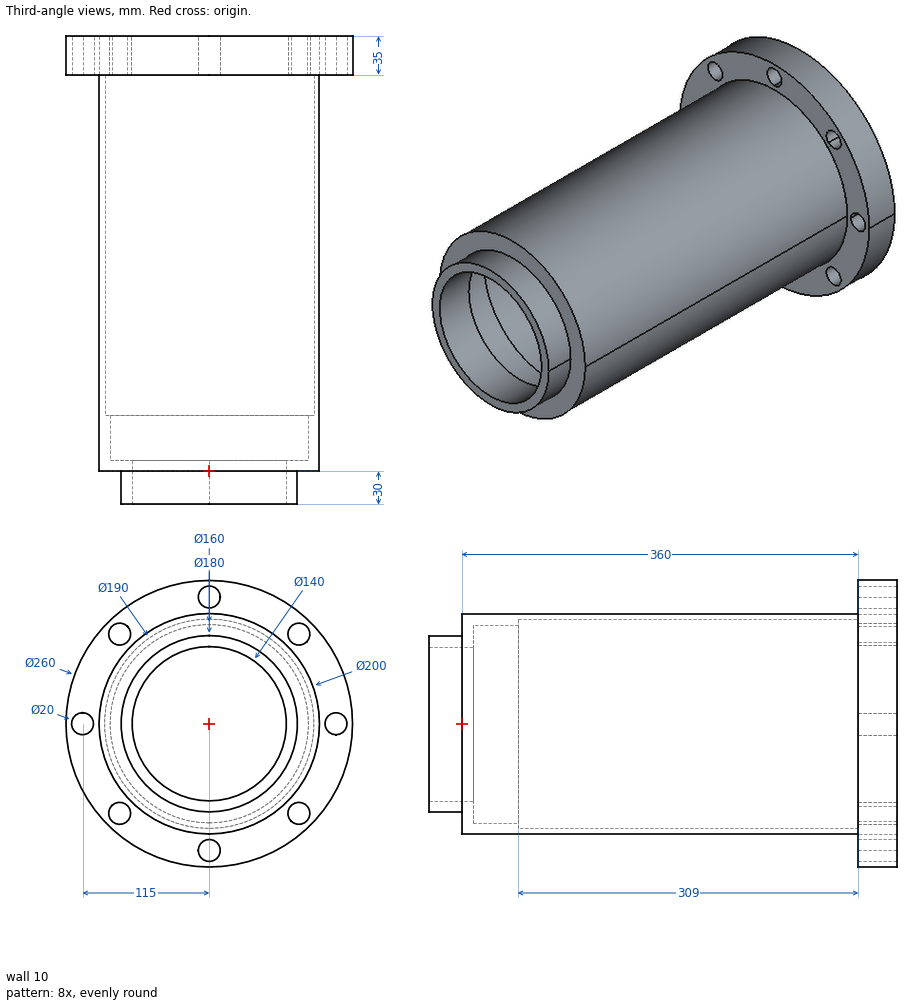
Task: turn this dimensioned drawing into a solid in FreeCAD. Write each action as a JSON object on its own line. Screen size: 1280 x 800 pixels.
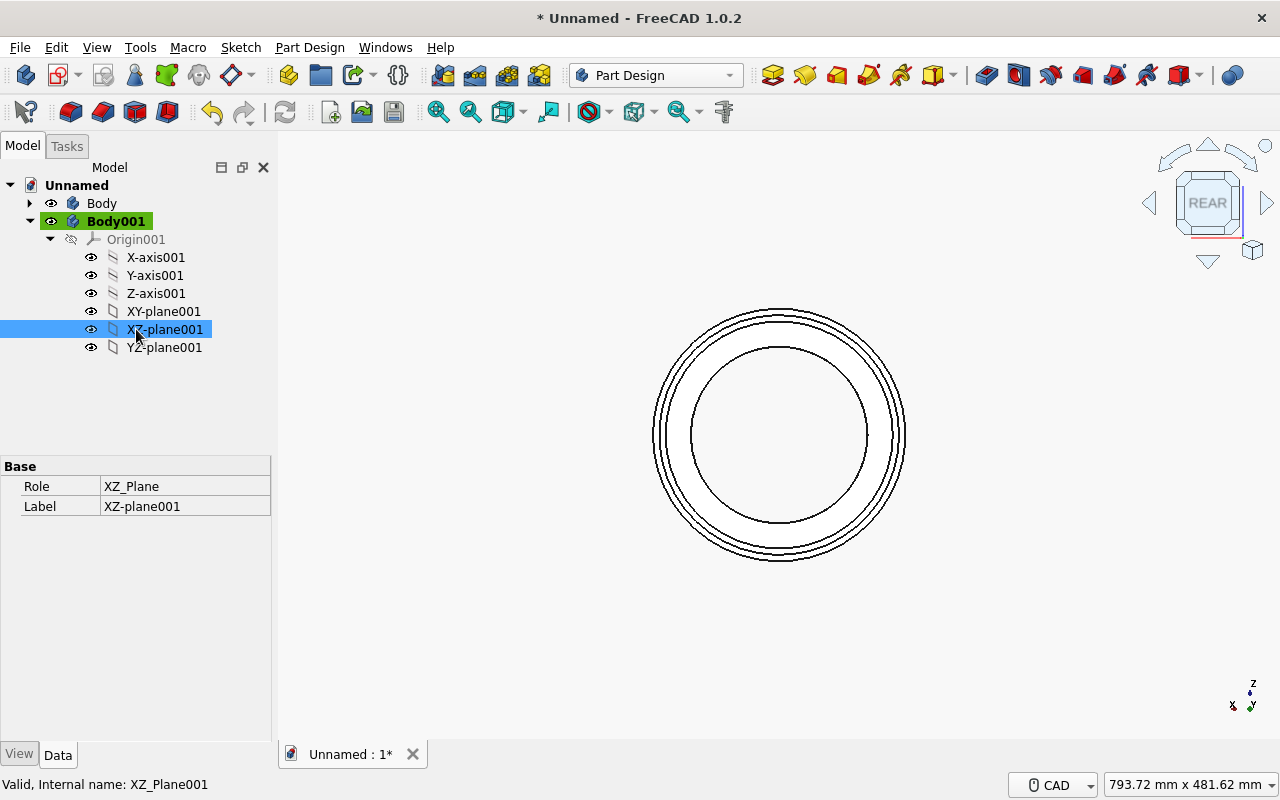
{"action": "left_click", "coordinate": [232, 76]}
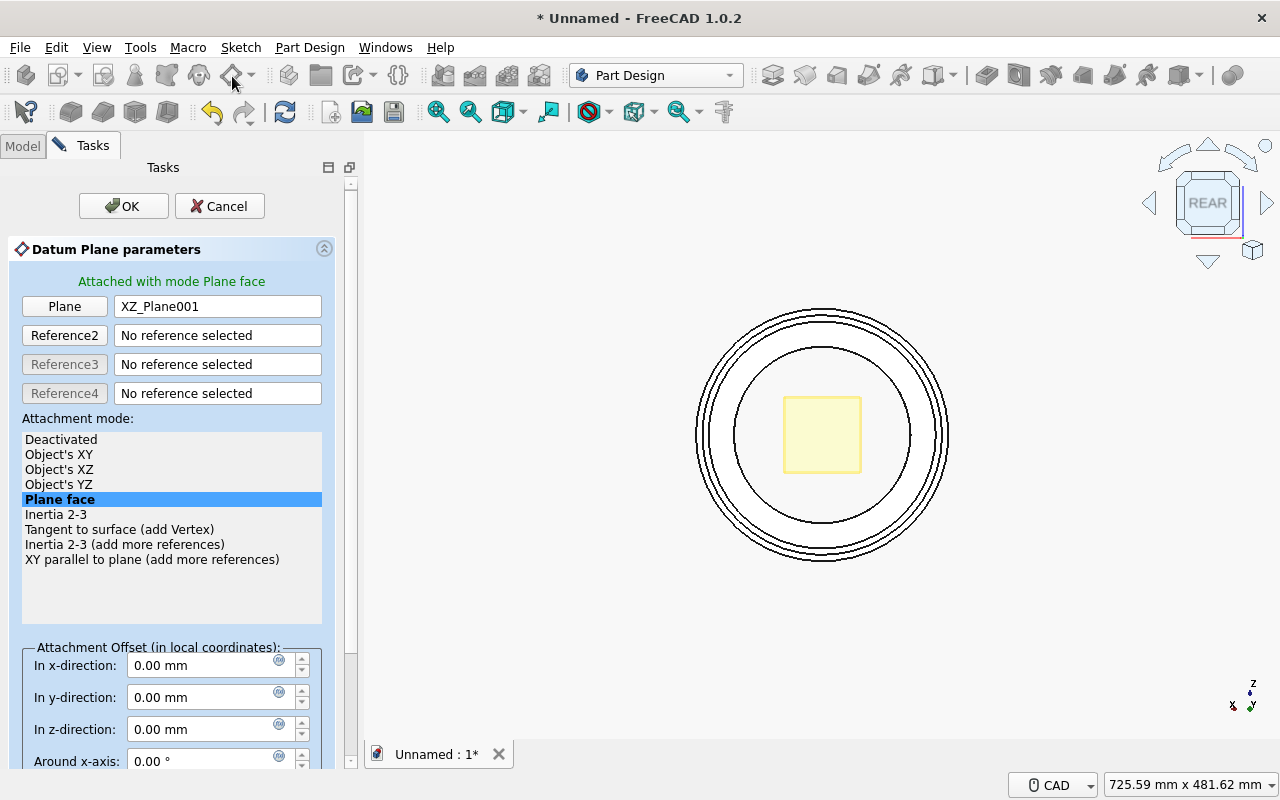
{"action": "triple_click", "coordinate": [210, 729]}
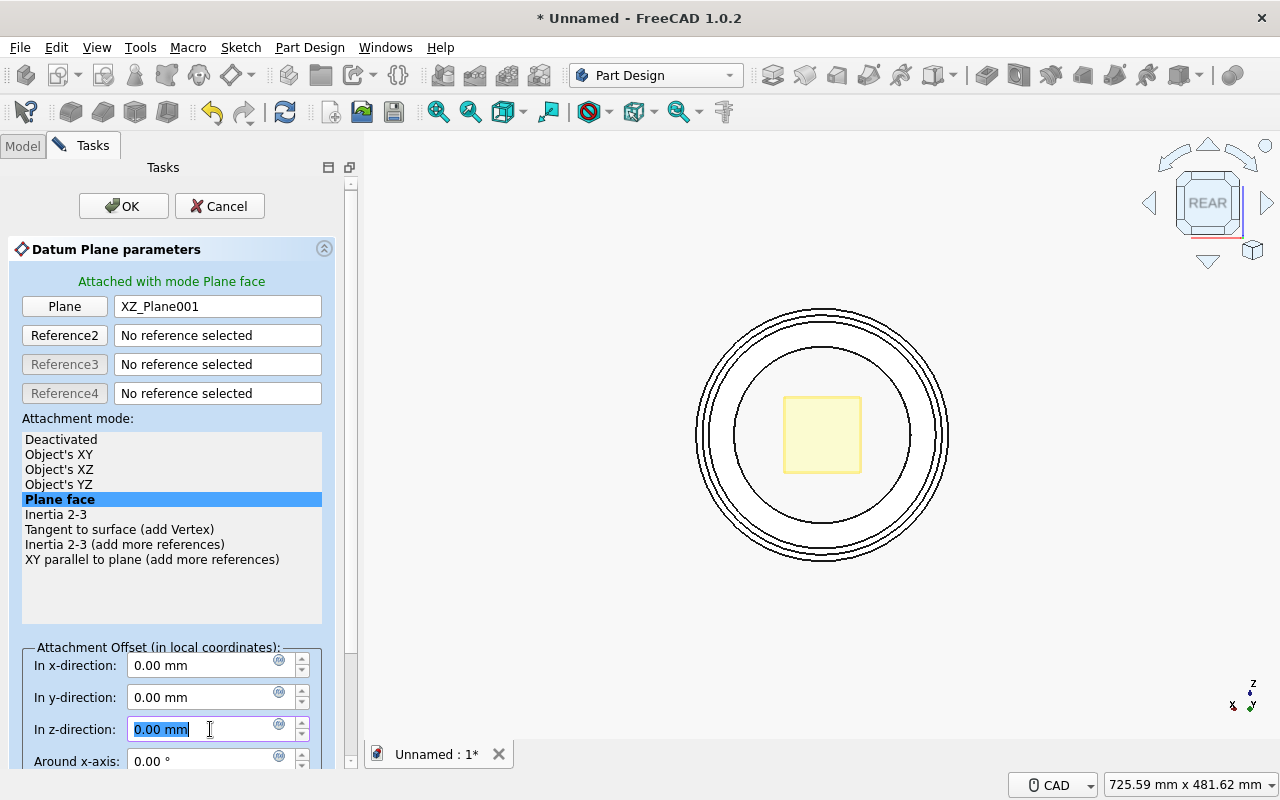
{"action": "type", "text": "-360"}
{"action": "key", "text": "Tab"}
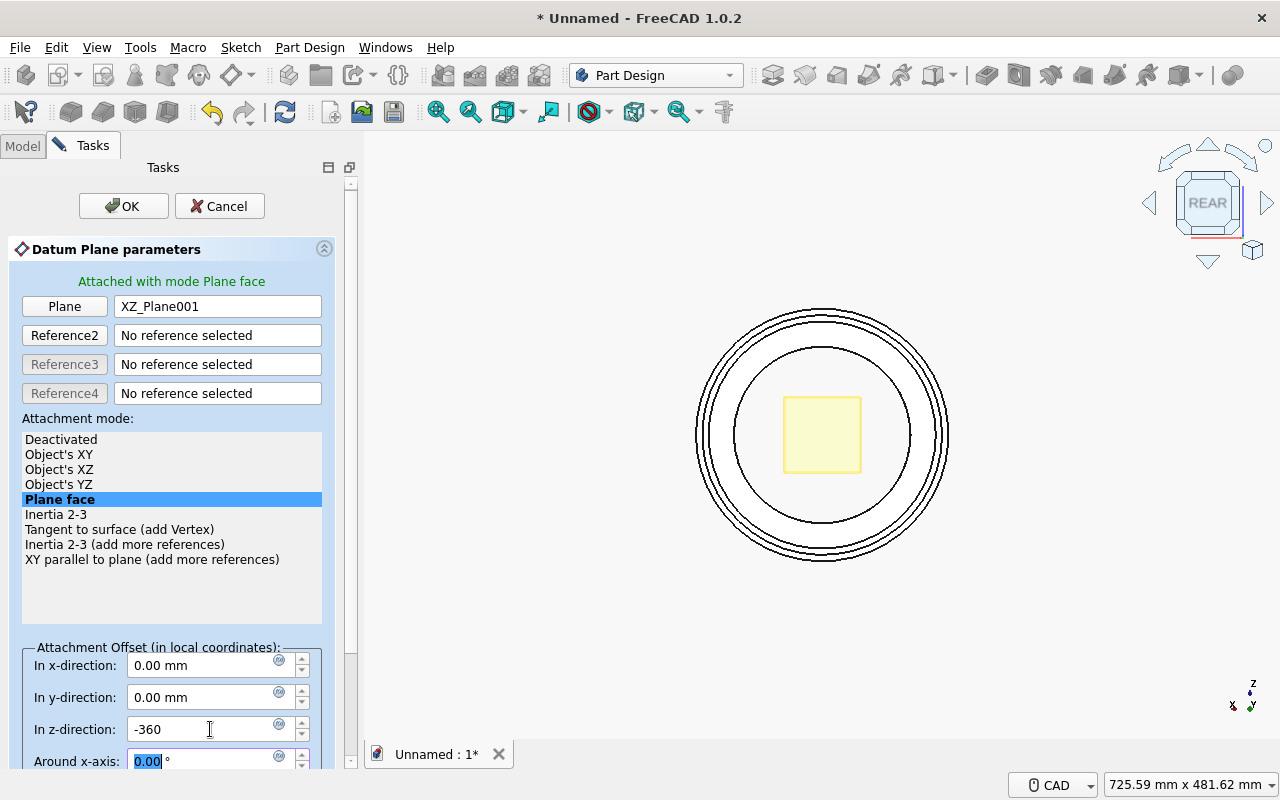
{"action": "left_click", "coordinate": [124, 206]}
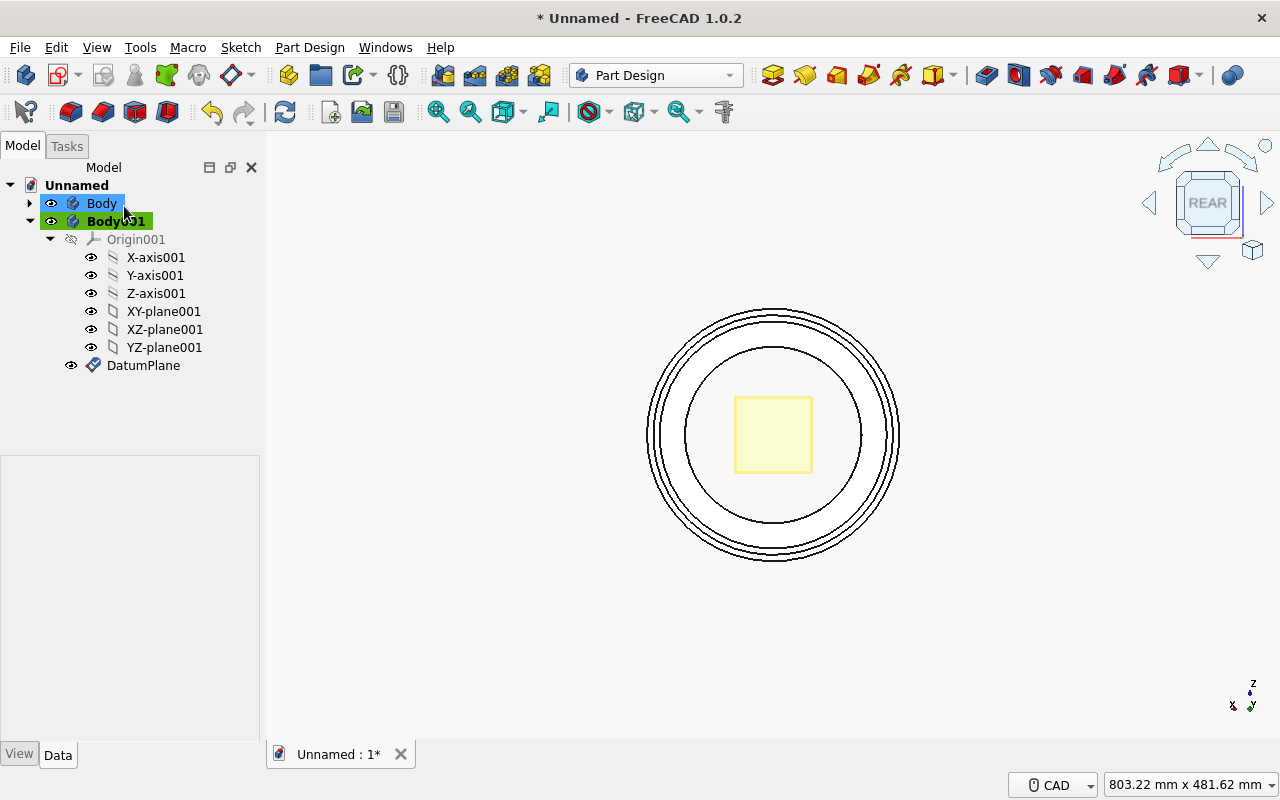
{"action": "left_click", "coordinate": [116, 365]}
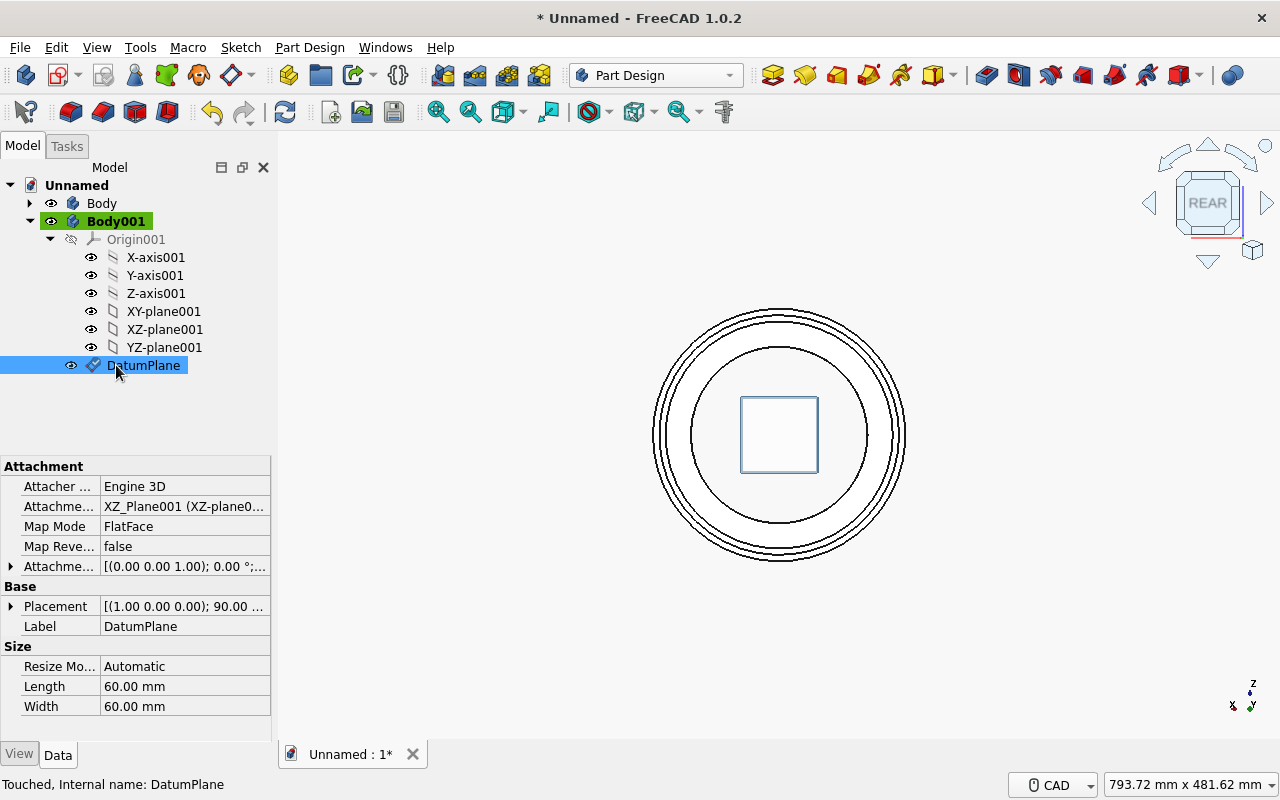
{"action": "left_click", "coordinate": [58, 76]}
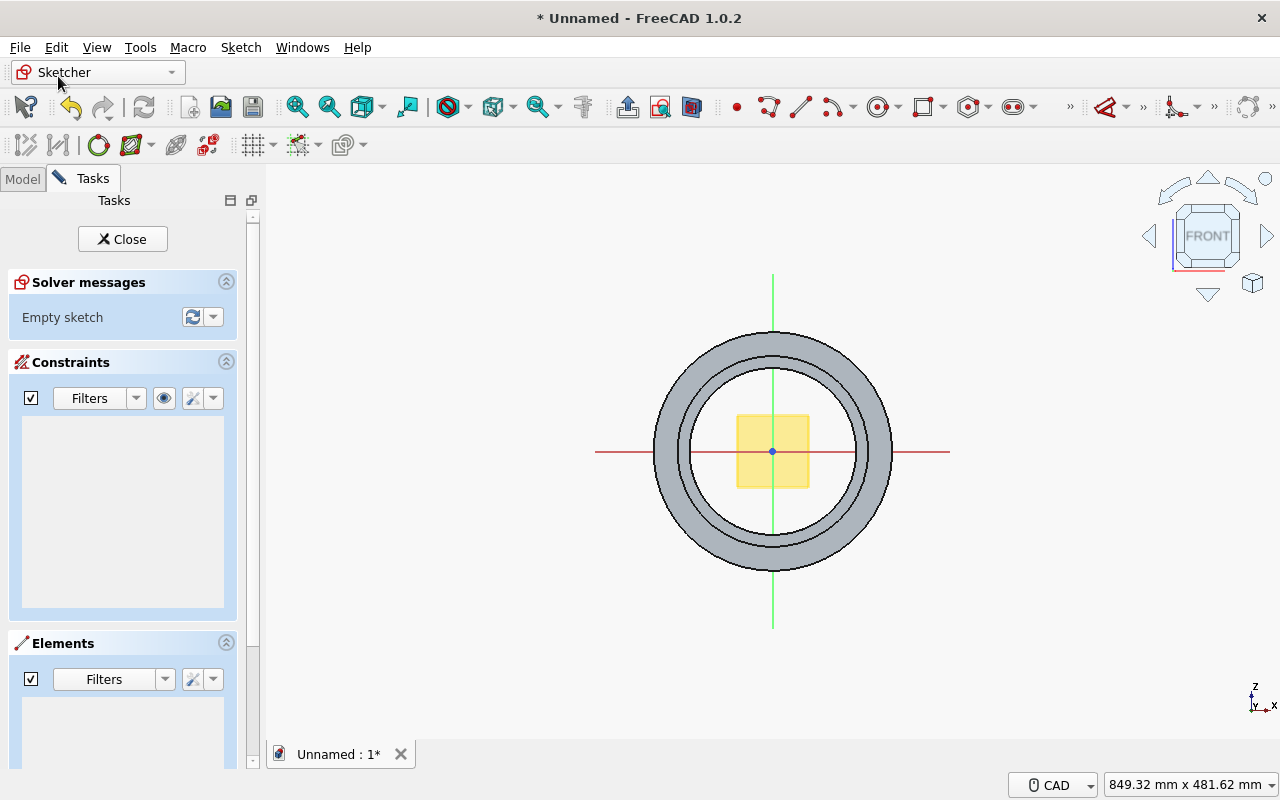
{"action": "left_click", "coordinate": [878, 108]}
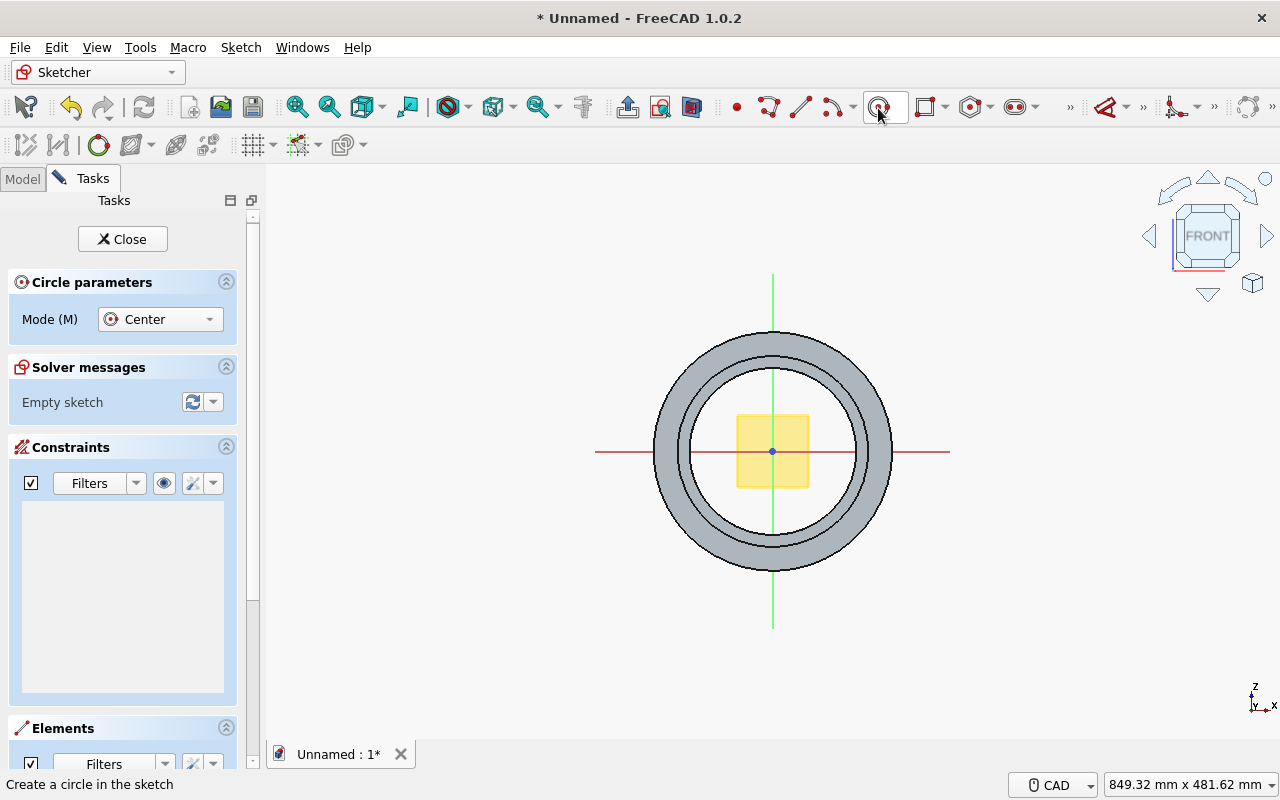
{"action": "left_click", "coordinate": [773, 452]}
{"action": "left_click", "coordinate": [883, 342]}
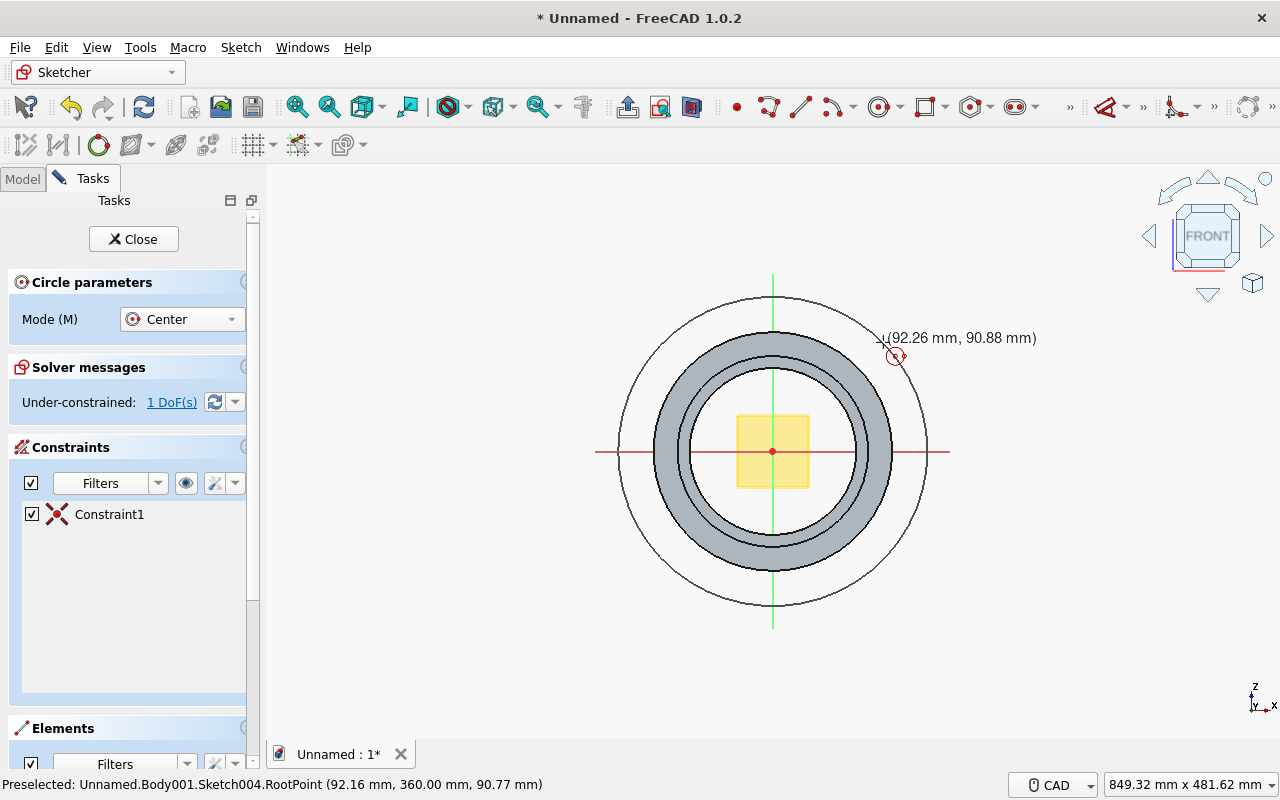
{"action": "left_click", "coordinate": [773, 452]}
{"action": "left_click", "coordinate": [857, 367]}
{"action": "key", "text": "Escape"}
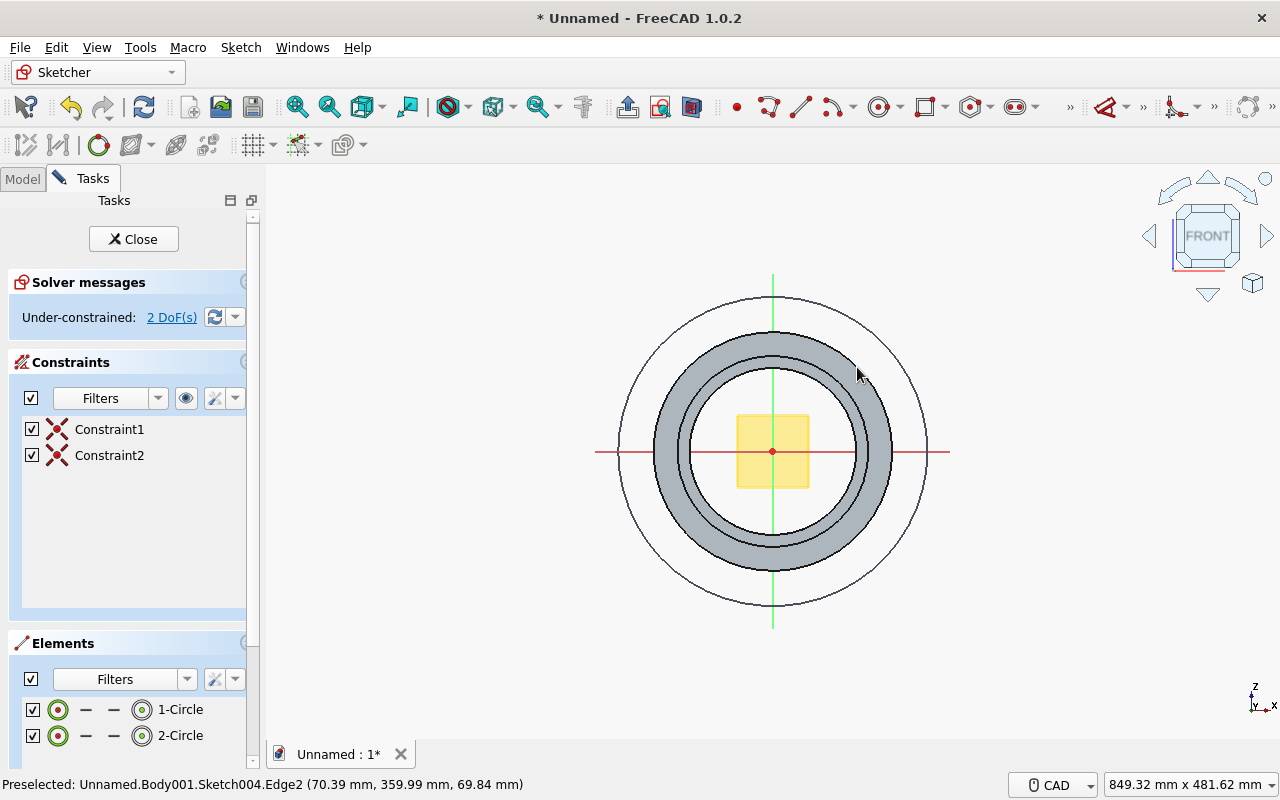
{"action": "left_click", "coordinate": [1106, 108]}